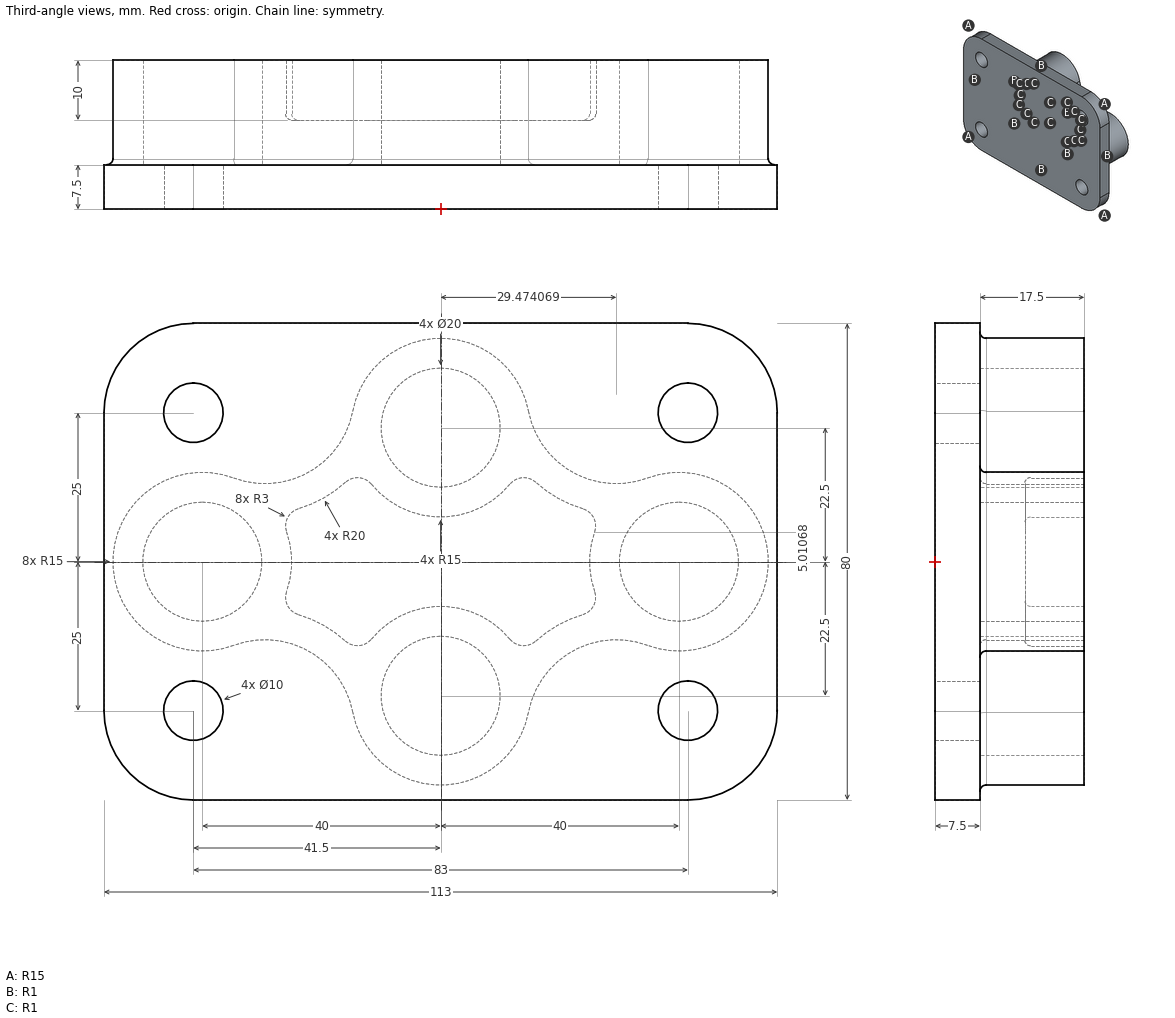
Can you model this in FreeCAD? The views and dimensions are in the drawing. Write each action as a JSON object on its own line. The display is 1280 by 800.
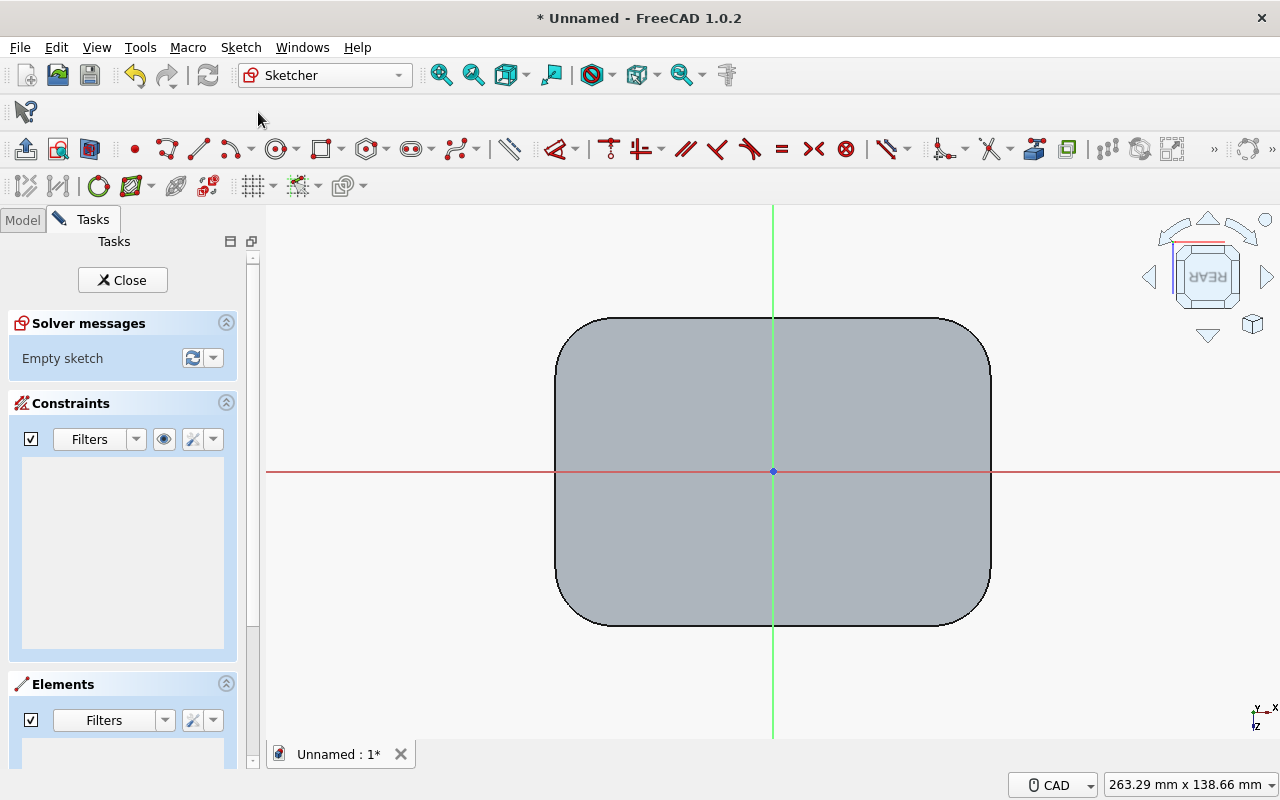
{"action": "scroll", "coordinate": [912, 472], "scroll_direction": "up", "scroll_amount": 2}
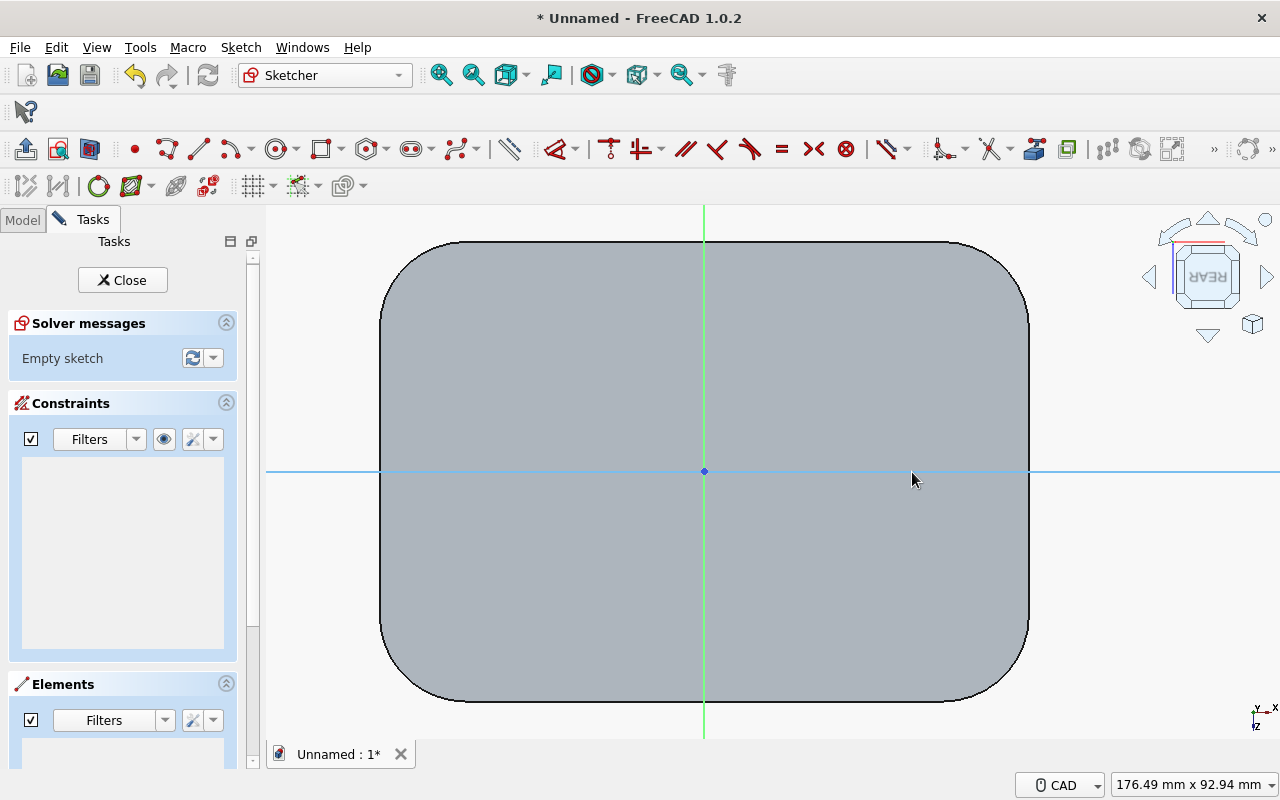
{"action": "key", "text": "g c"}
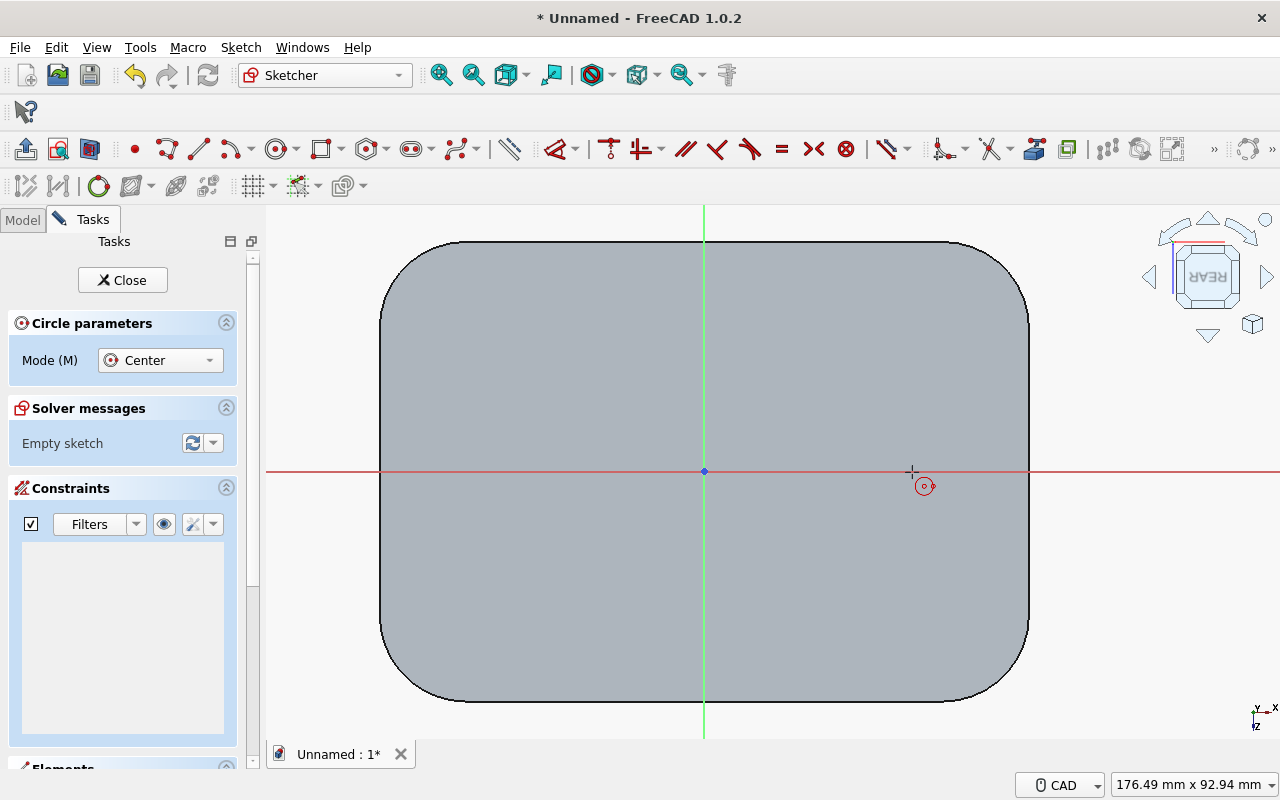
{"action": "left_click", "coordinate": [466, 328]}
{"action": "mouse_move", "coordinate": [486, 308]}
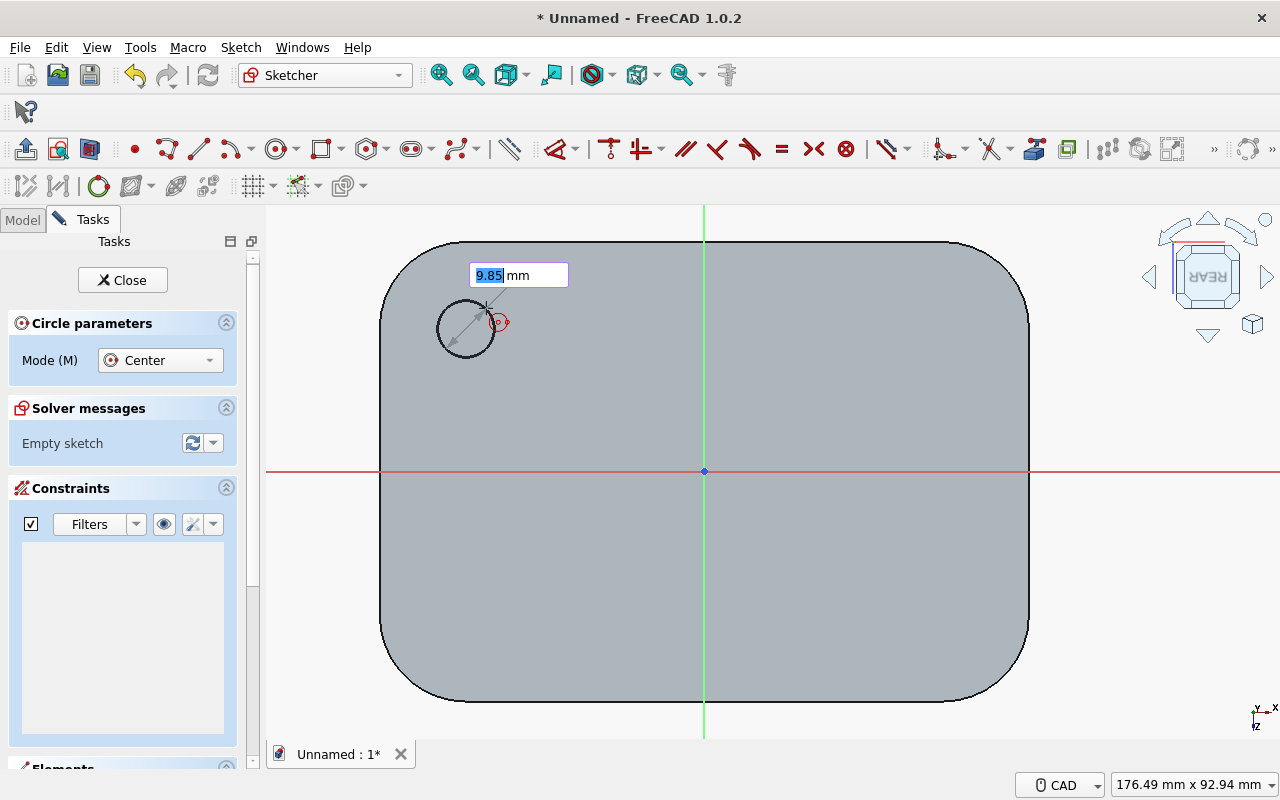
{"action": "type", "text": "10"}
{"action": "key", "text": "Return"}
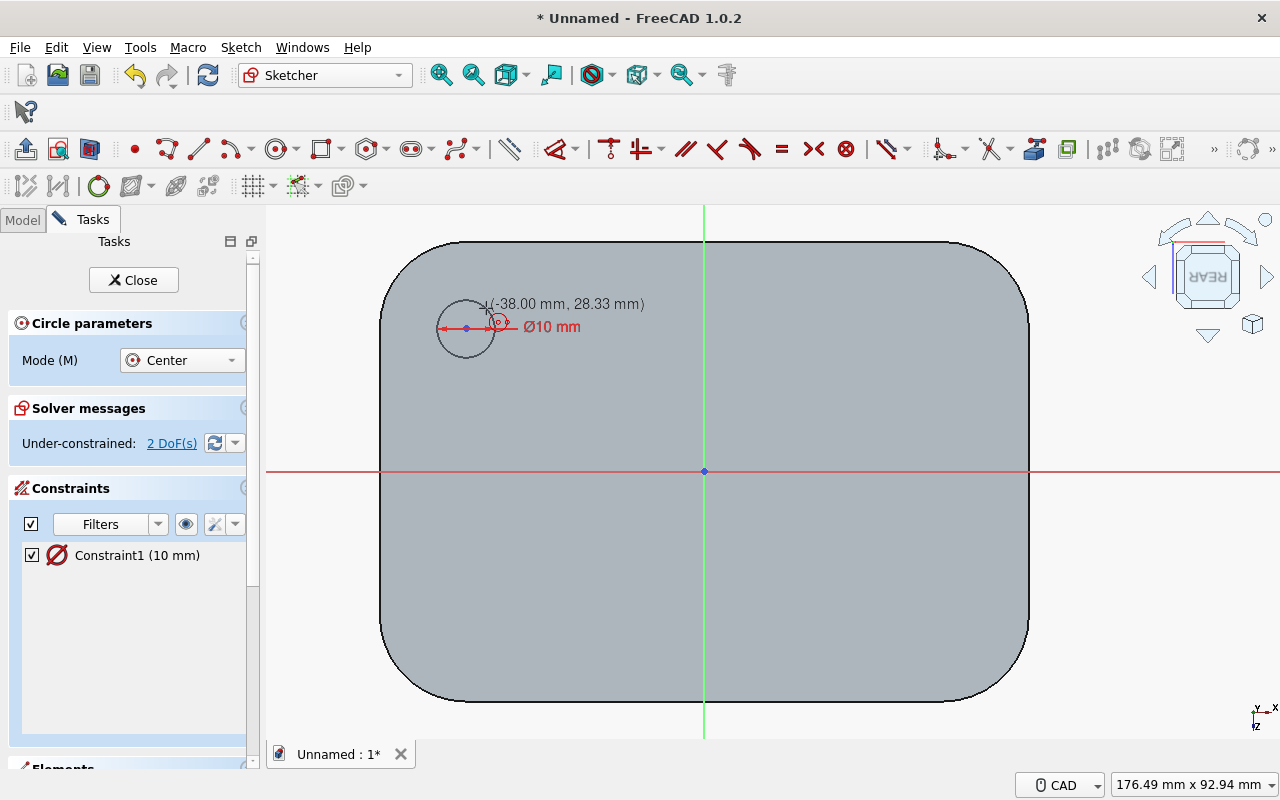
{"action": "left_click", "coordinate": [943, 328]}
{"action": "mouse_move", "coordinate": [963, 308]}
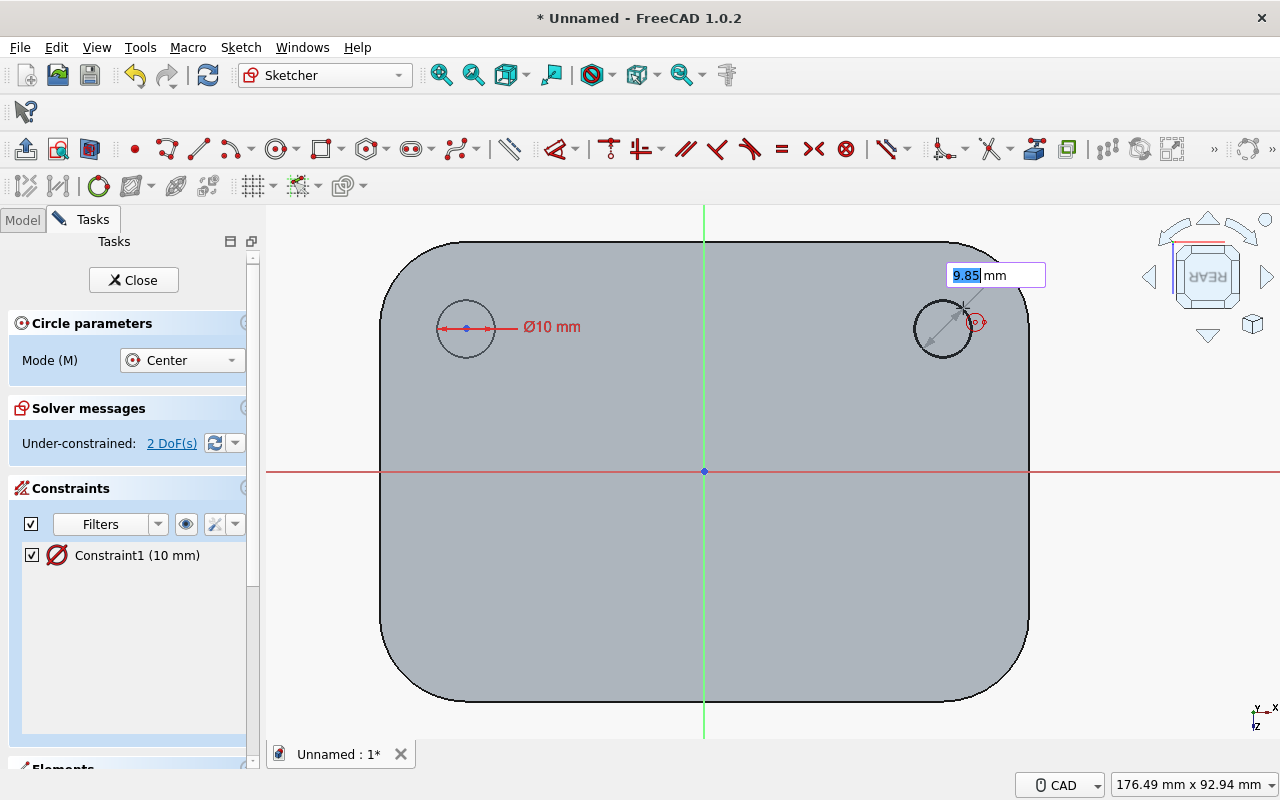
{"action": "type", "text": "10"}
{"action": "key", "text": "Return"}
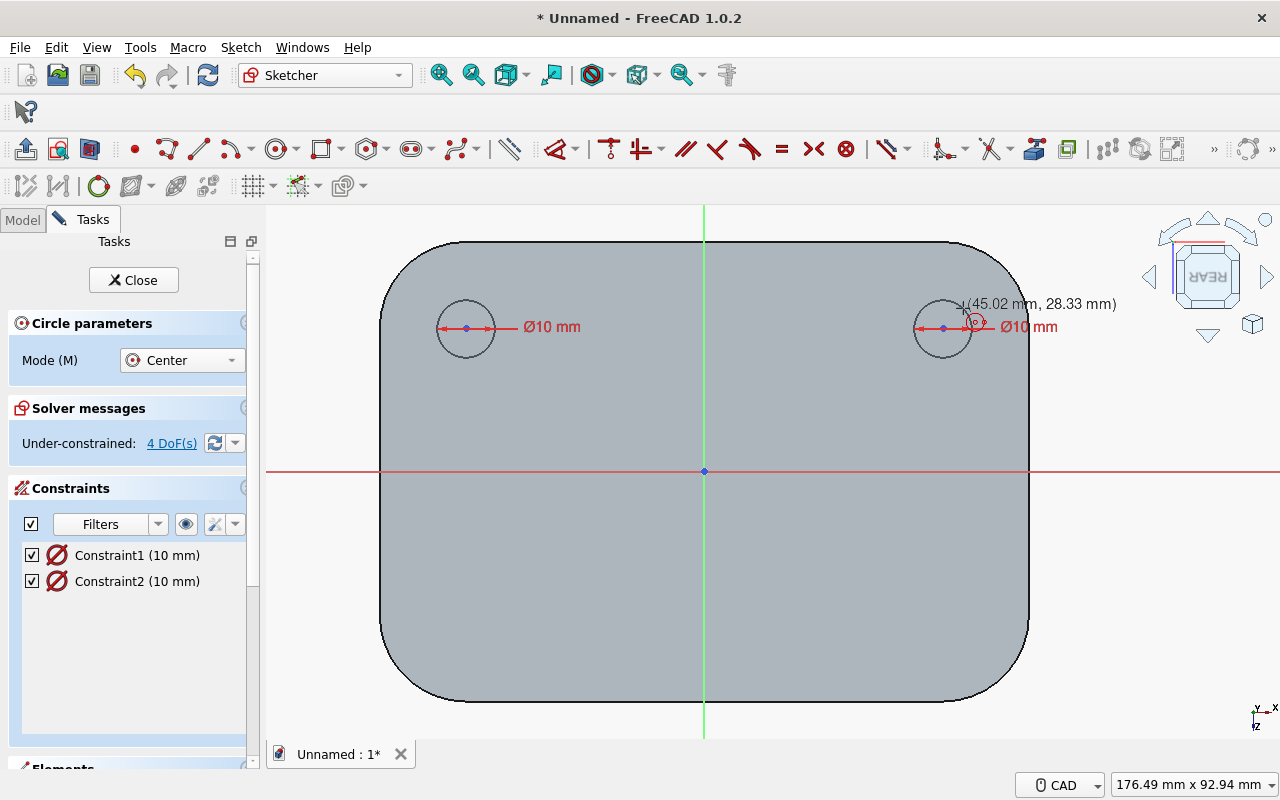
{"action": "left_click", "coordinate": [466, 615]}
{"action": "mouse_move", "coordinate": [486, 595]}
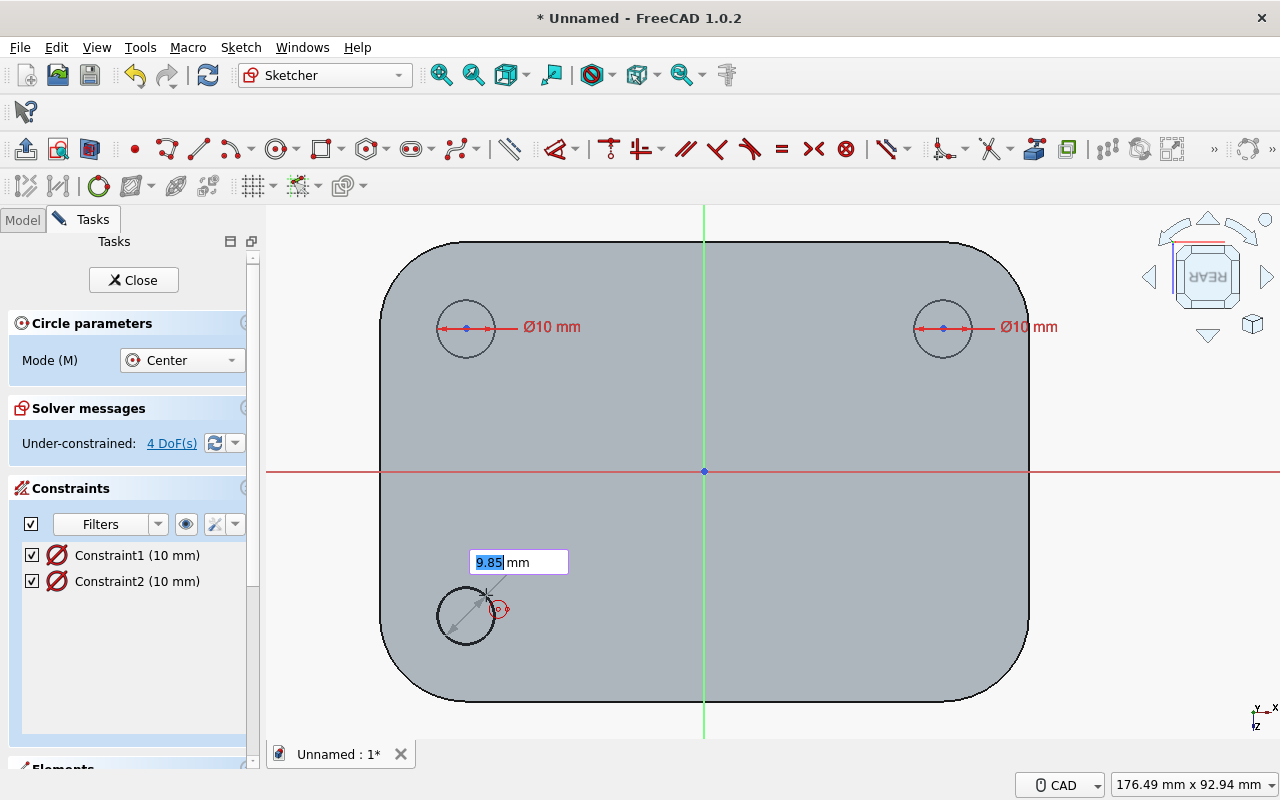
{"action": "type", "text": "10"}
{"action": "key", "text": "Return"}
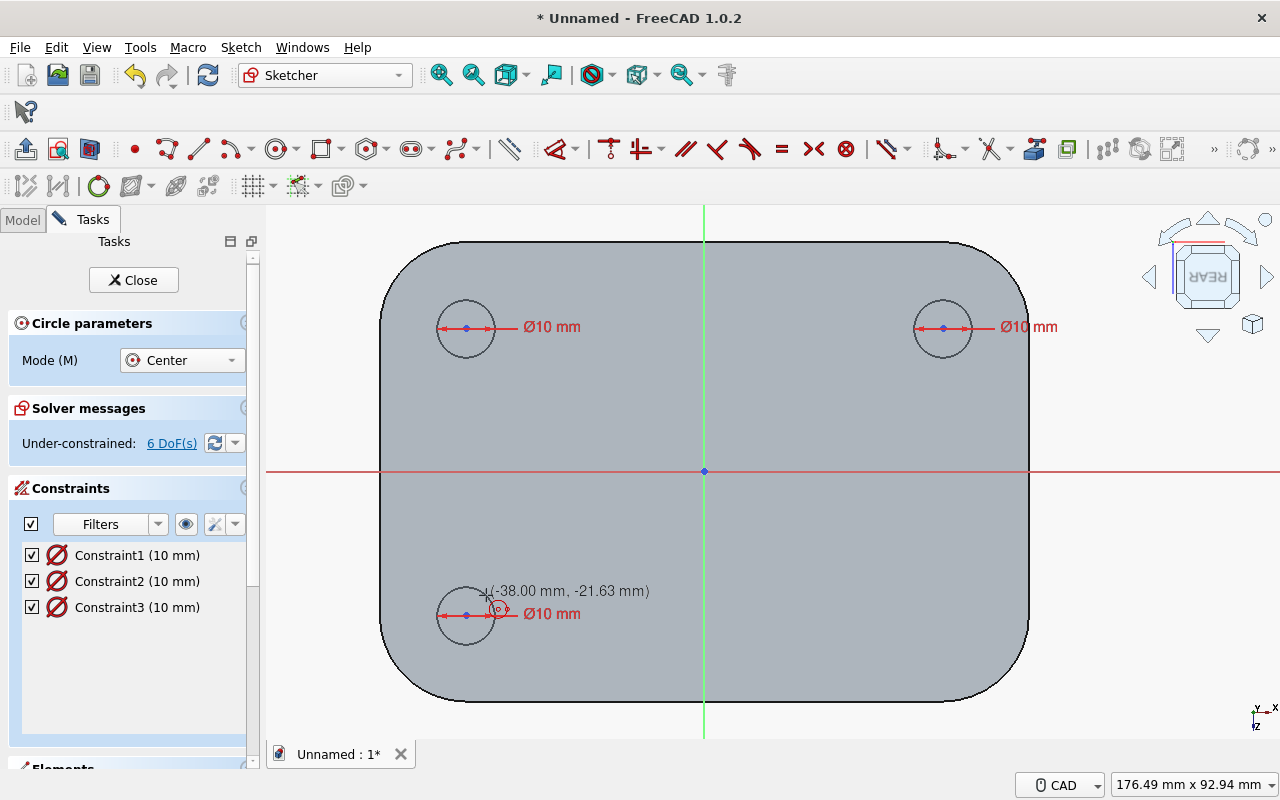
{"action": "left_click", "coordinate": [943, 615]}
{"action": "mouse_move", "coordinate": [963, 595]}